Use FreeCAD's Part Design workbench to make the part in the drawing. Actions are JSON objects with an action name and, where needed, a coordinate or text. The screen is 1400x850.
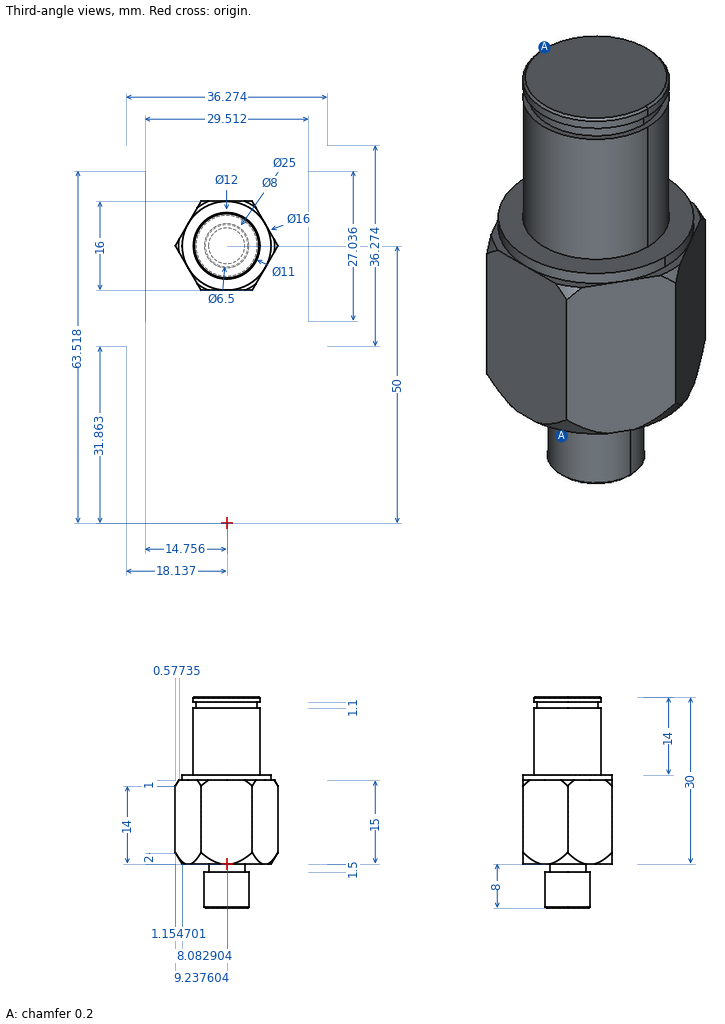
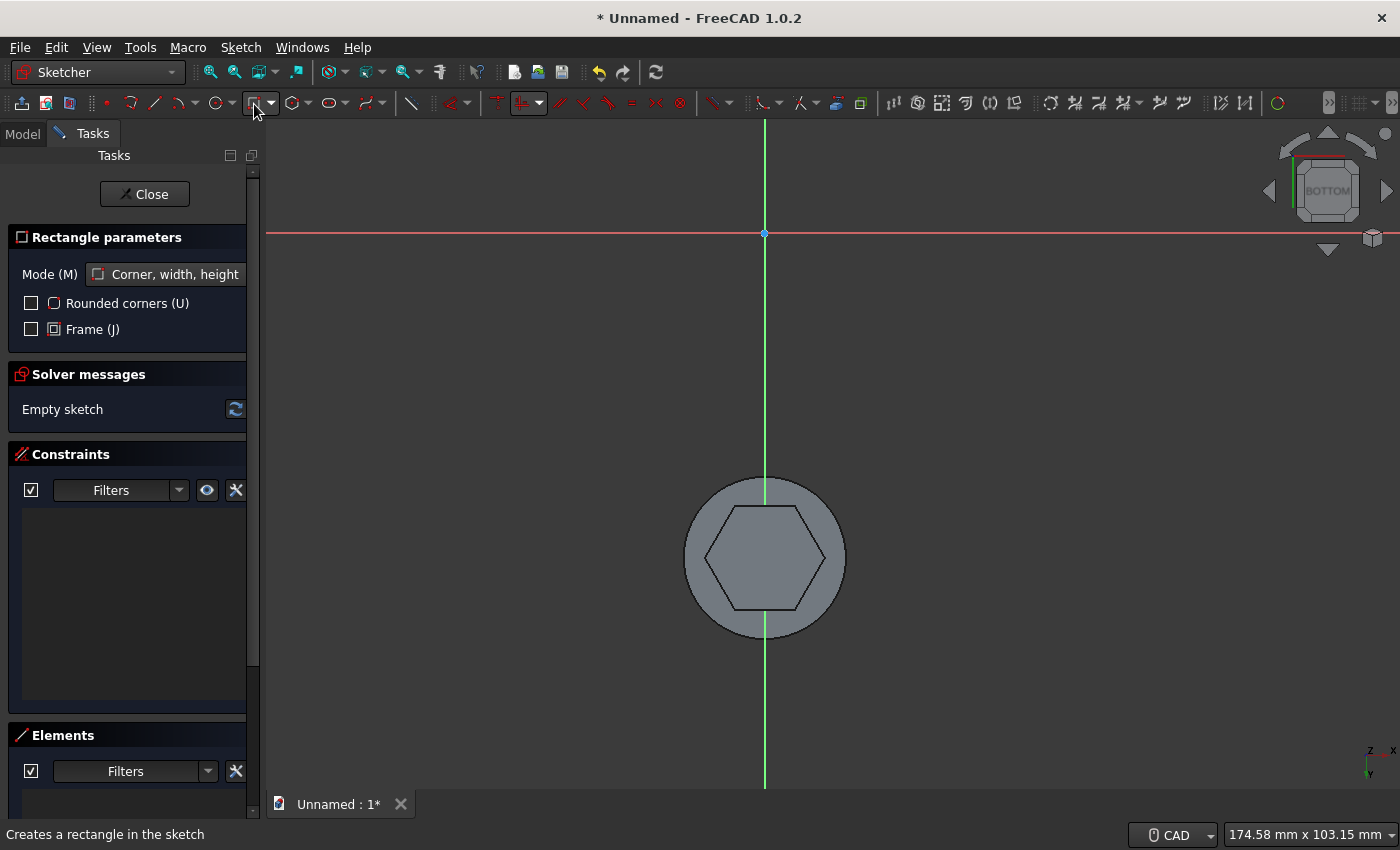
{"action": "left_click", "coordinate": [647, 440]}
{"action": "mouse_move", "coordinate": [883, 676]}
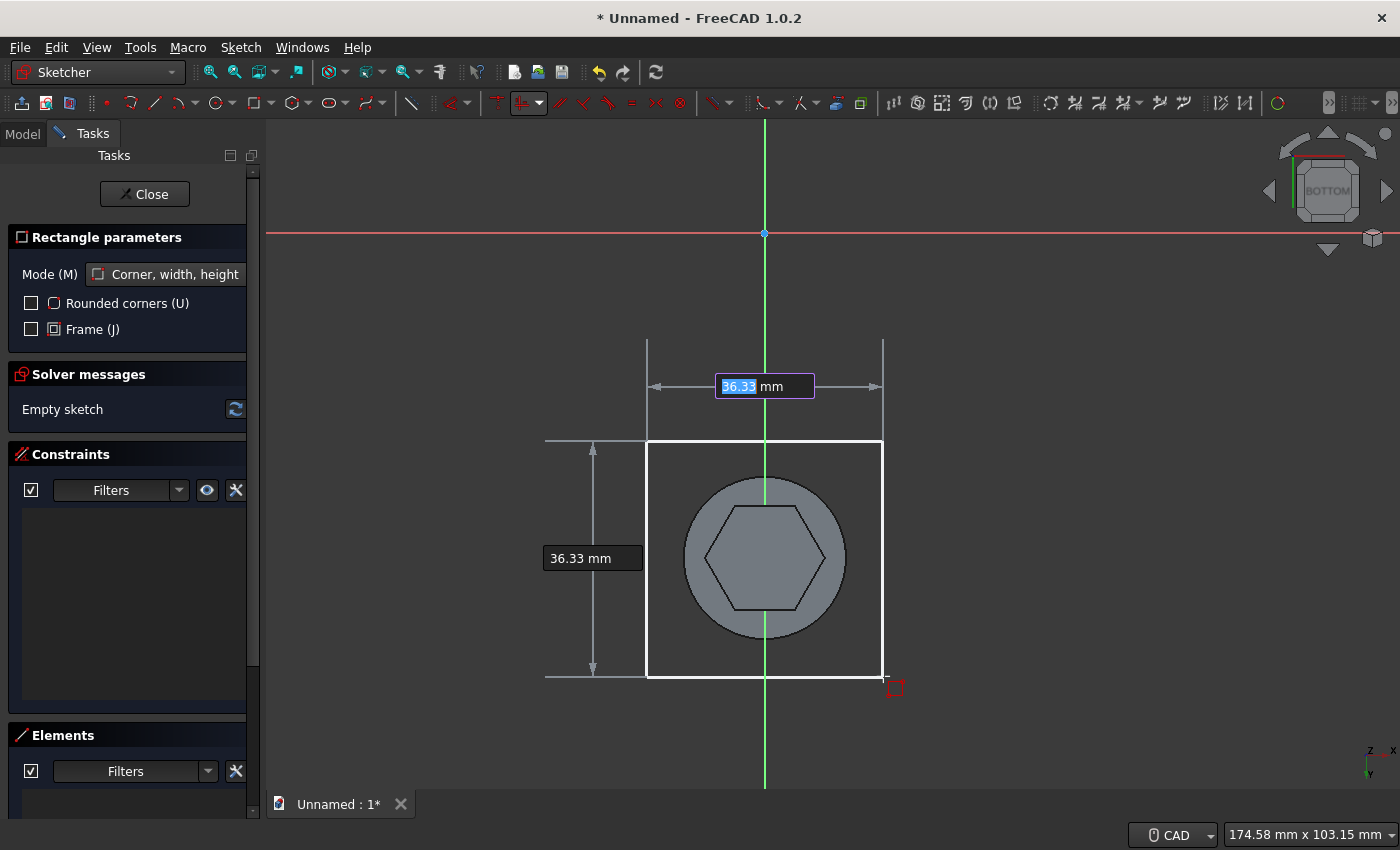
{"action": "type", "text": "36.274"}
{"action": "key", "text": "Tab"}
{"action": "type", "text": "36.274"}
{"action": "key", "text": "Return"}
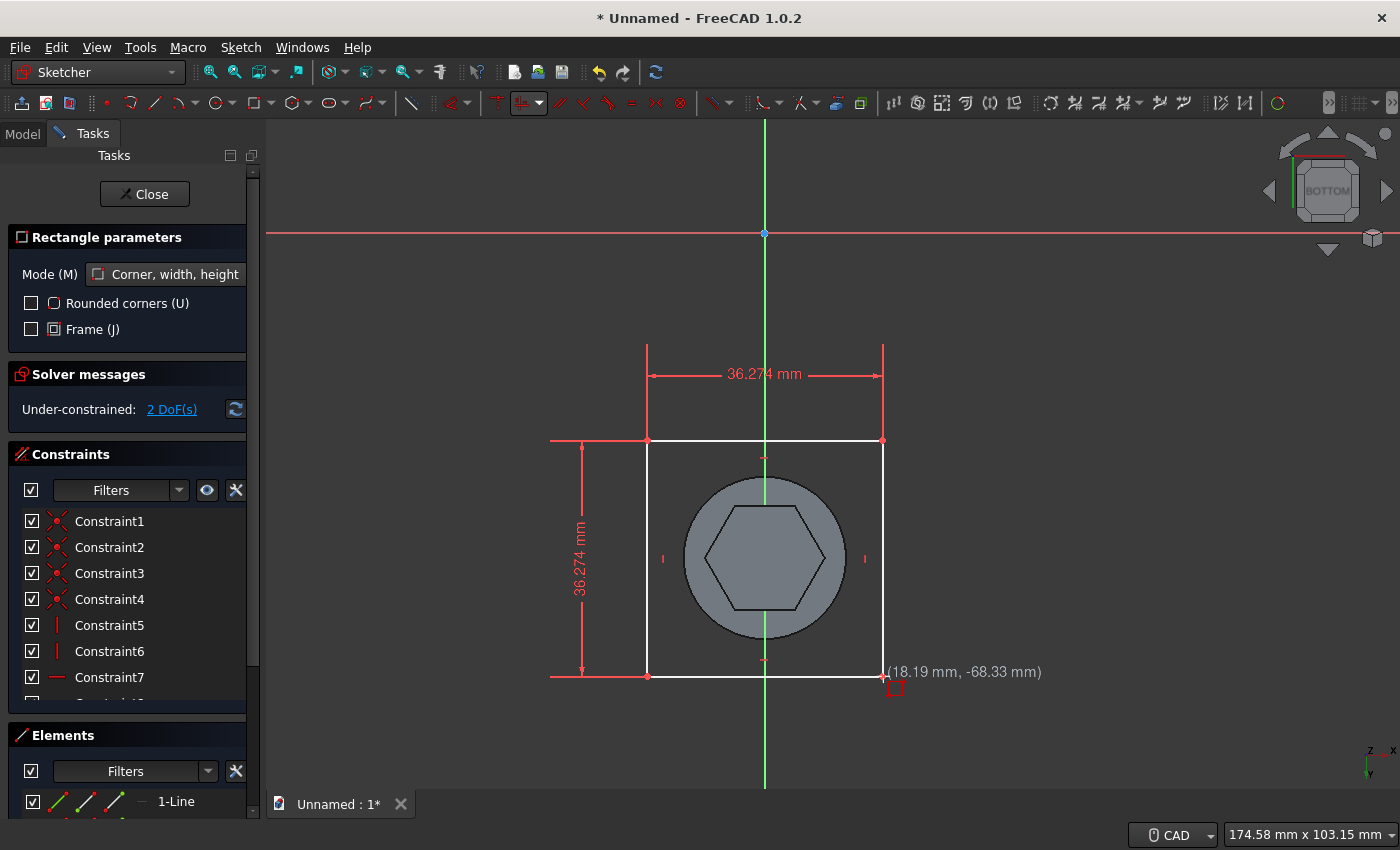
{"action": "left_click", "coordinate": [216, 104]}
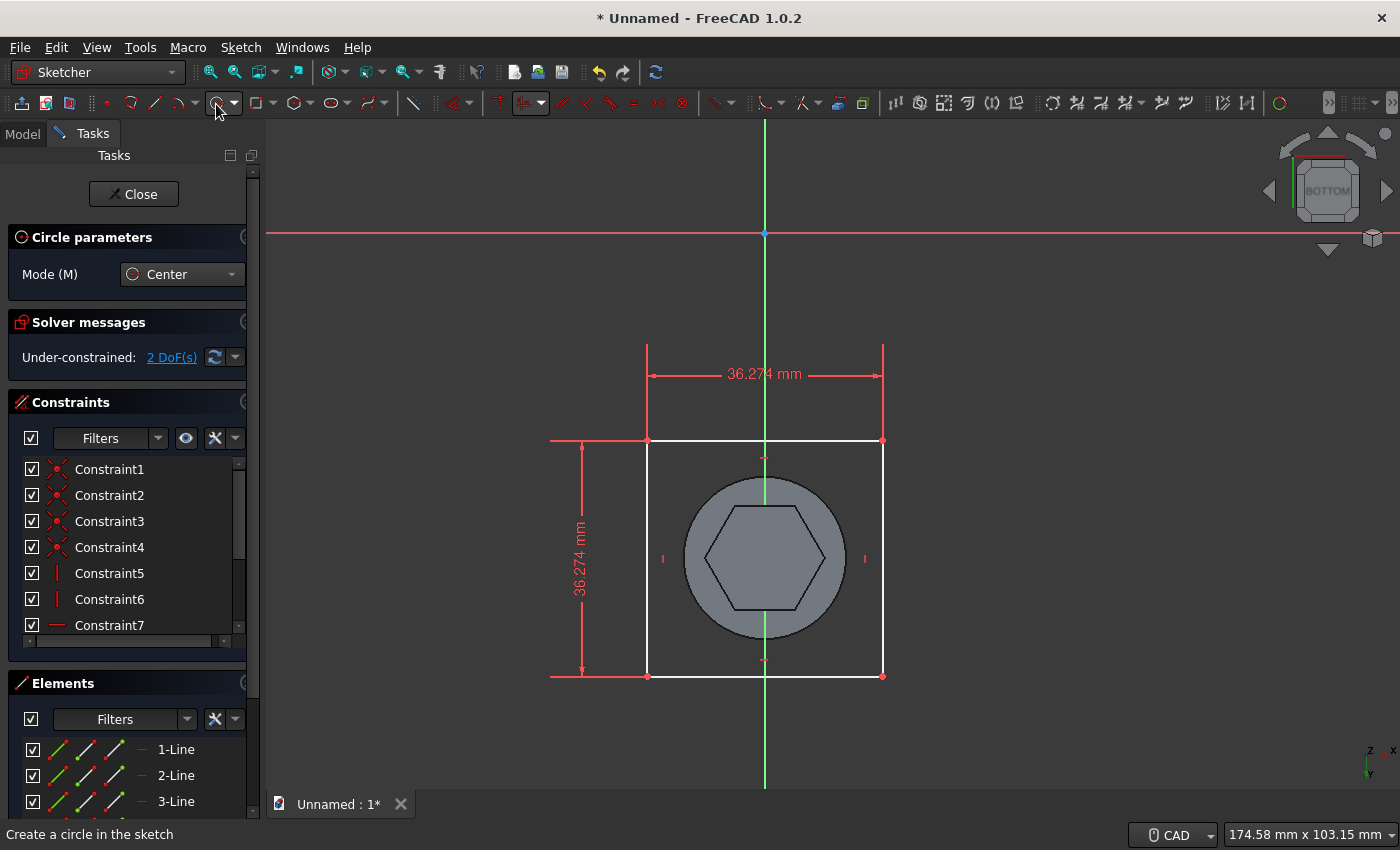
{"action": "left_click", "coordinate": [765, 558]}
{"action": "mouse_move", "coordinate": [802, 521]}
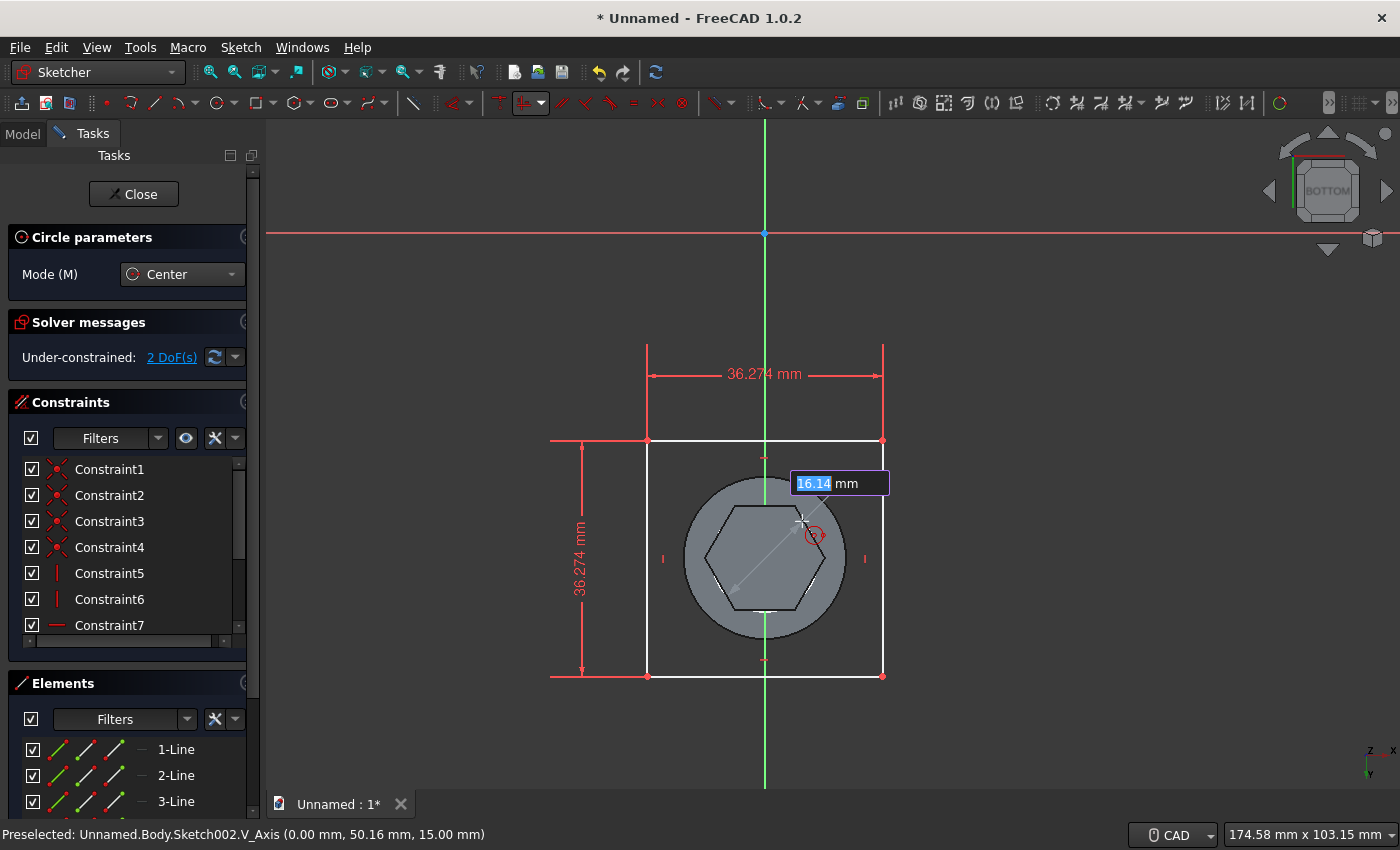
{"action": "type", "text": "16"}
{"action": "key", "text": "Return"}
{"action": "key", "text": "Escape"}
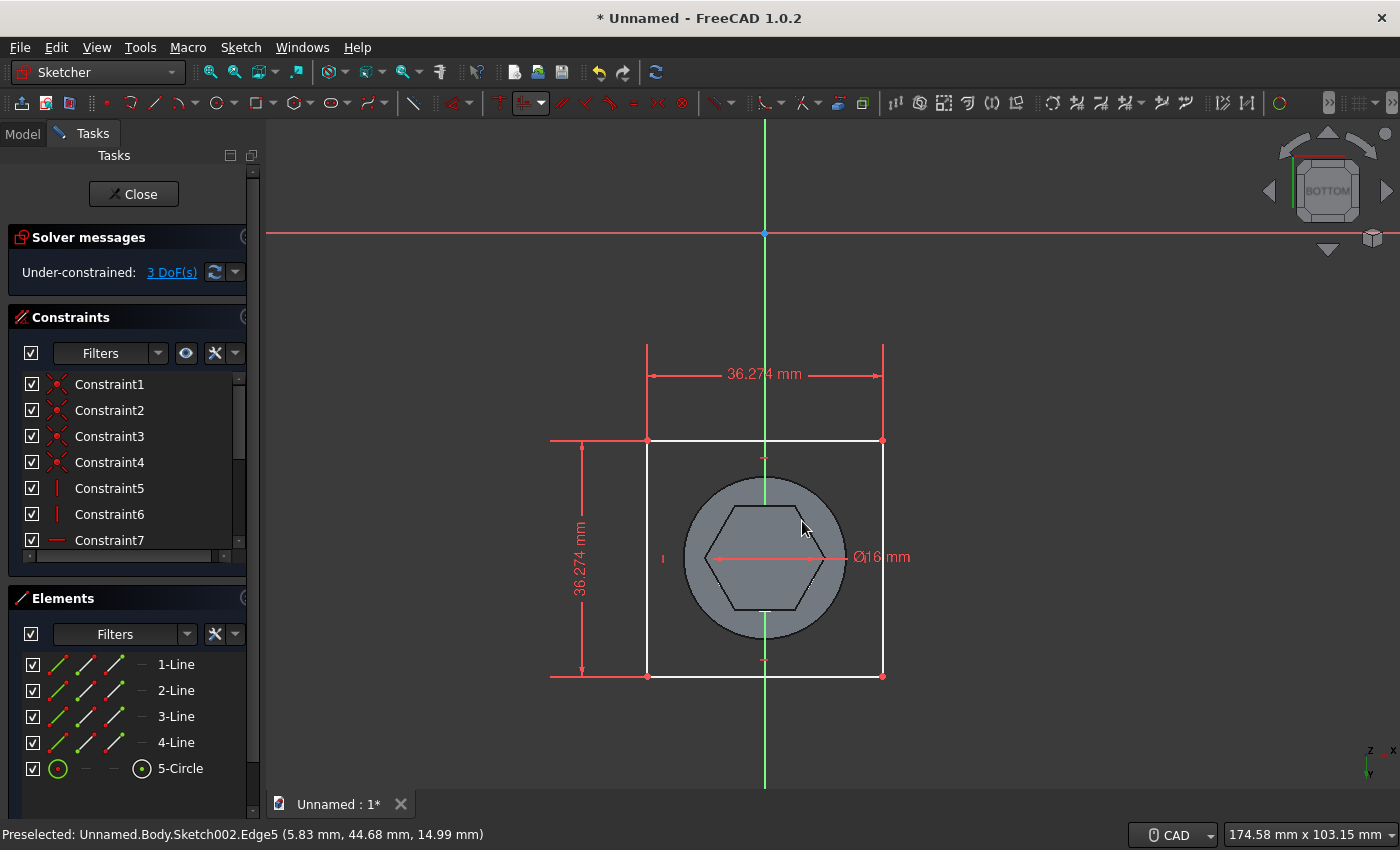
{"action": "left_click", "coordinate": [452, 104]}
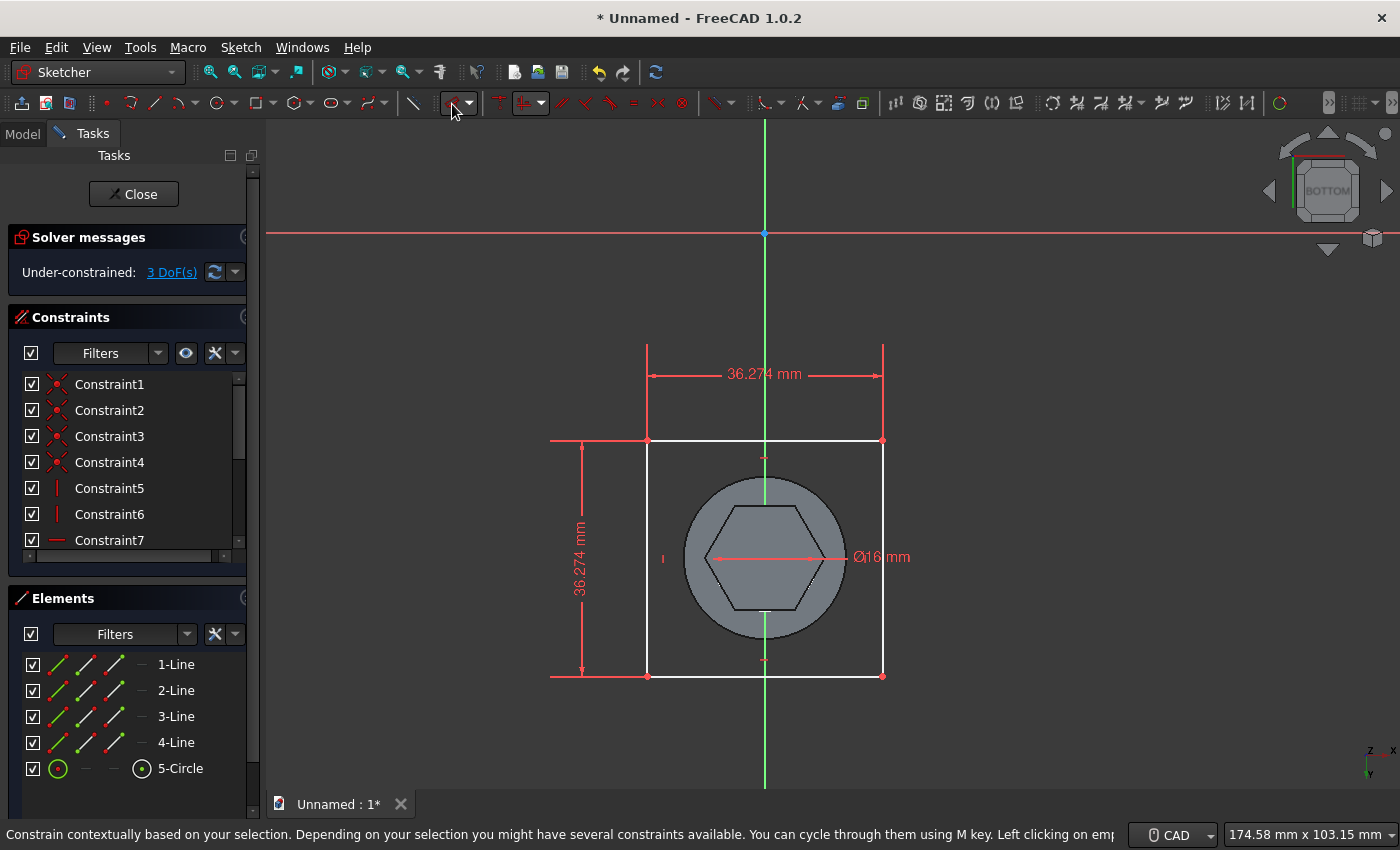
{"action": "left_click", "coordinate": [765, 559]}
{"action": "left_click", "coordinate": [799, 396]}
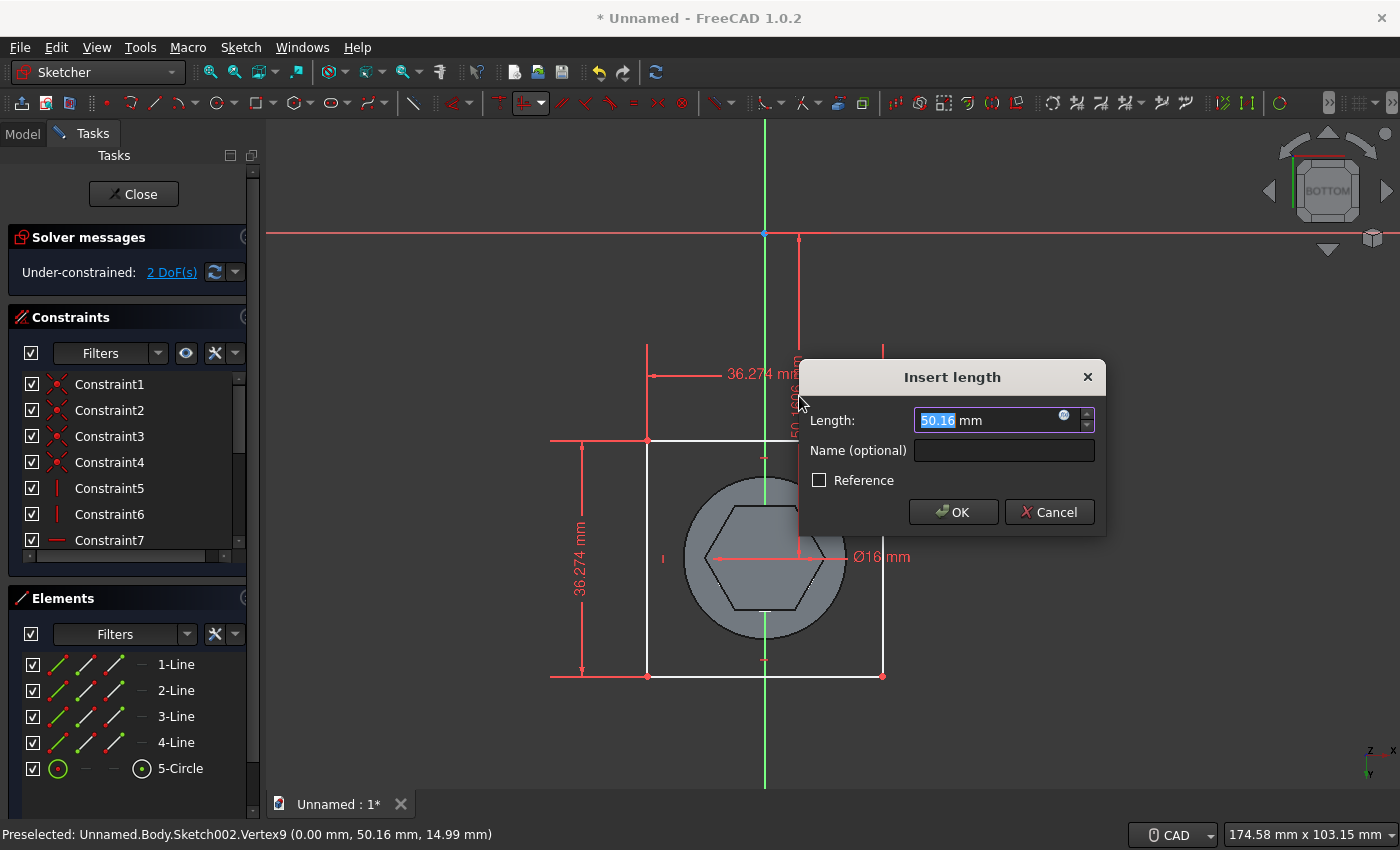
{"action": "type", "text": "50"}
{"action": "key", "text": "Return"}